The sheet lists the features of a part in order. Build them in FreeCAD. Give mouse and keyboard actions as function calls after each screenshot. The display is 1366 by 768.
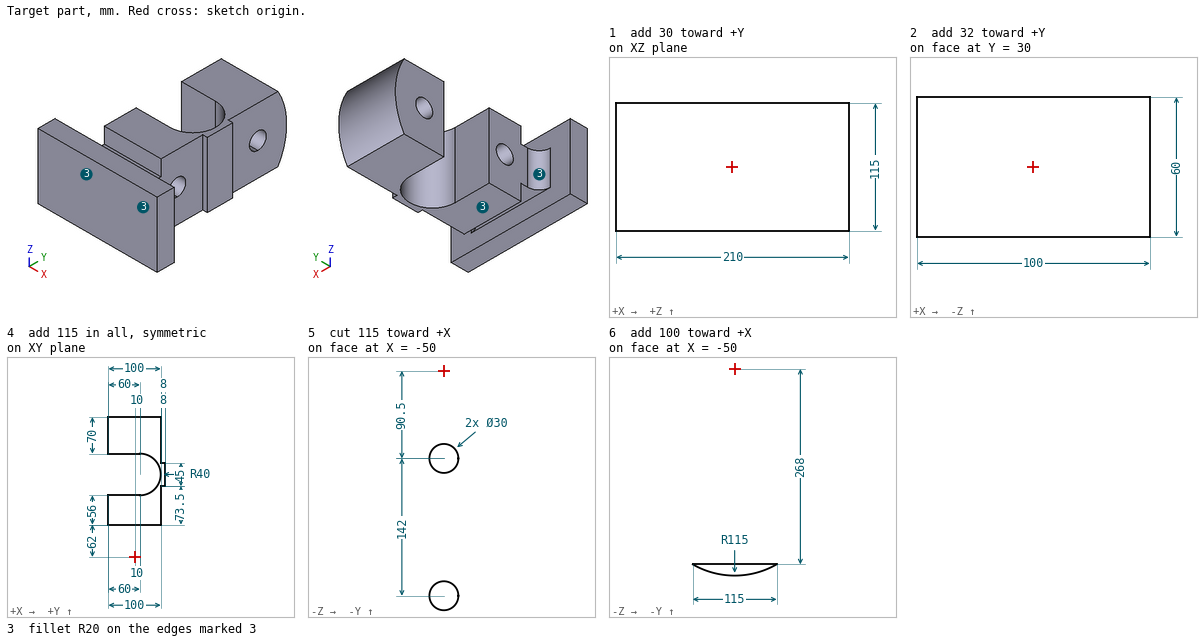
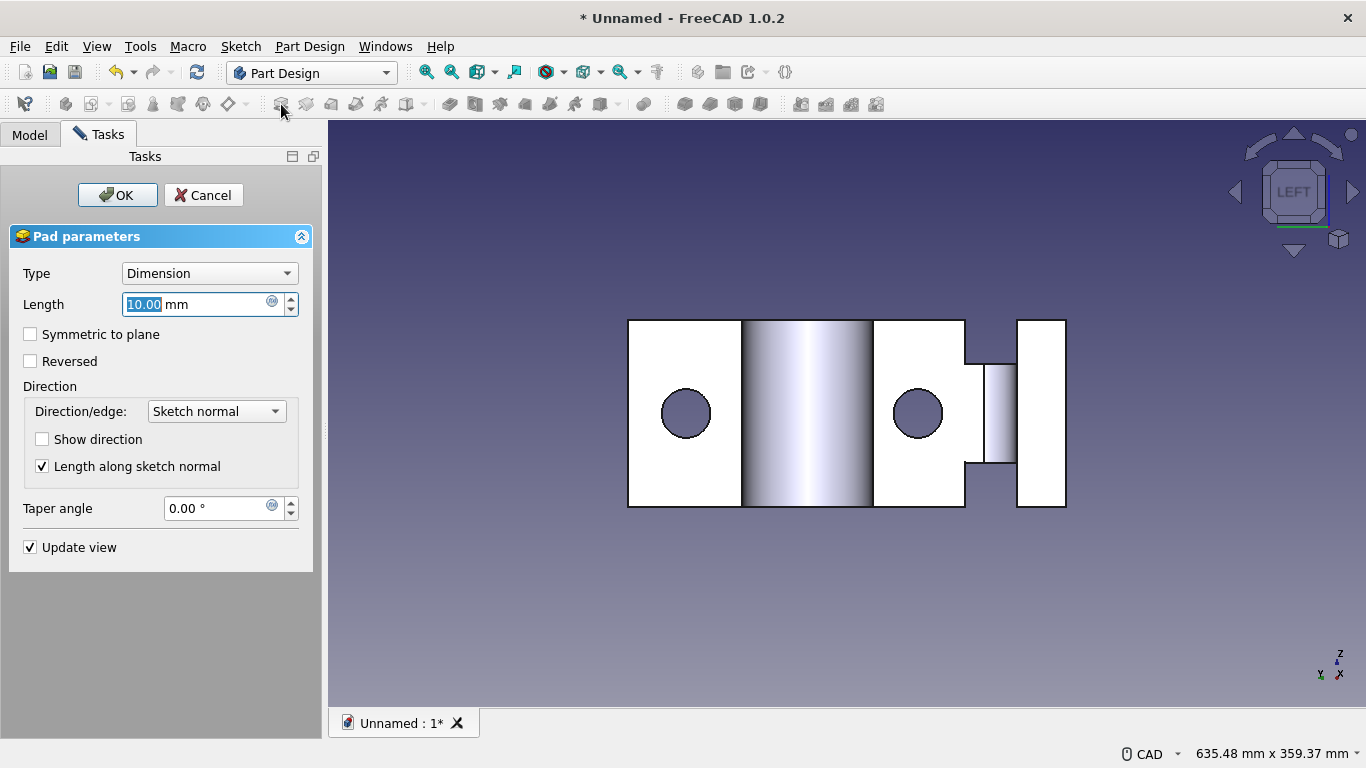
text(100)
key(Tab)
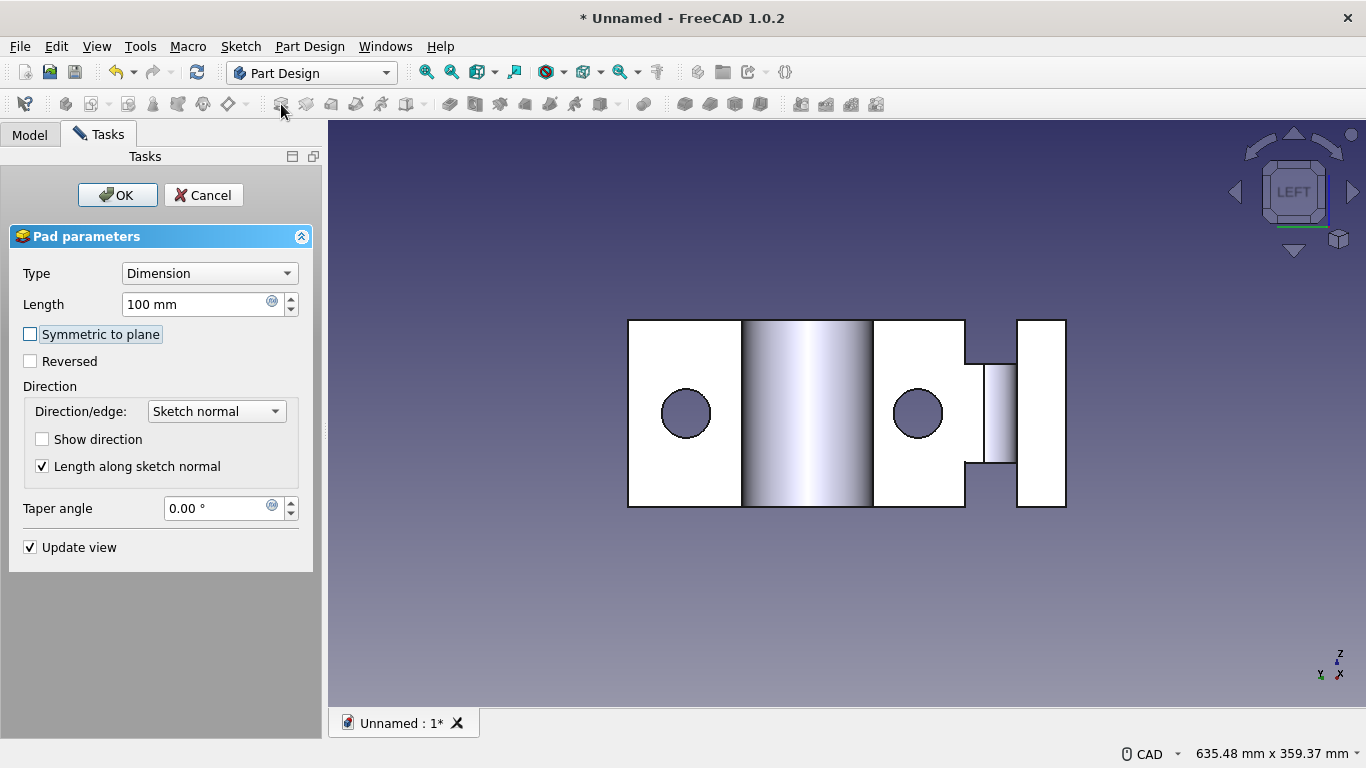
click(31, 361)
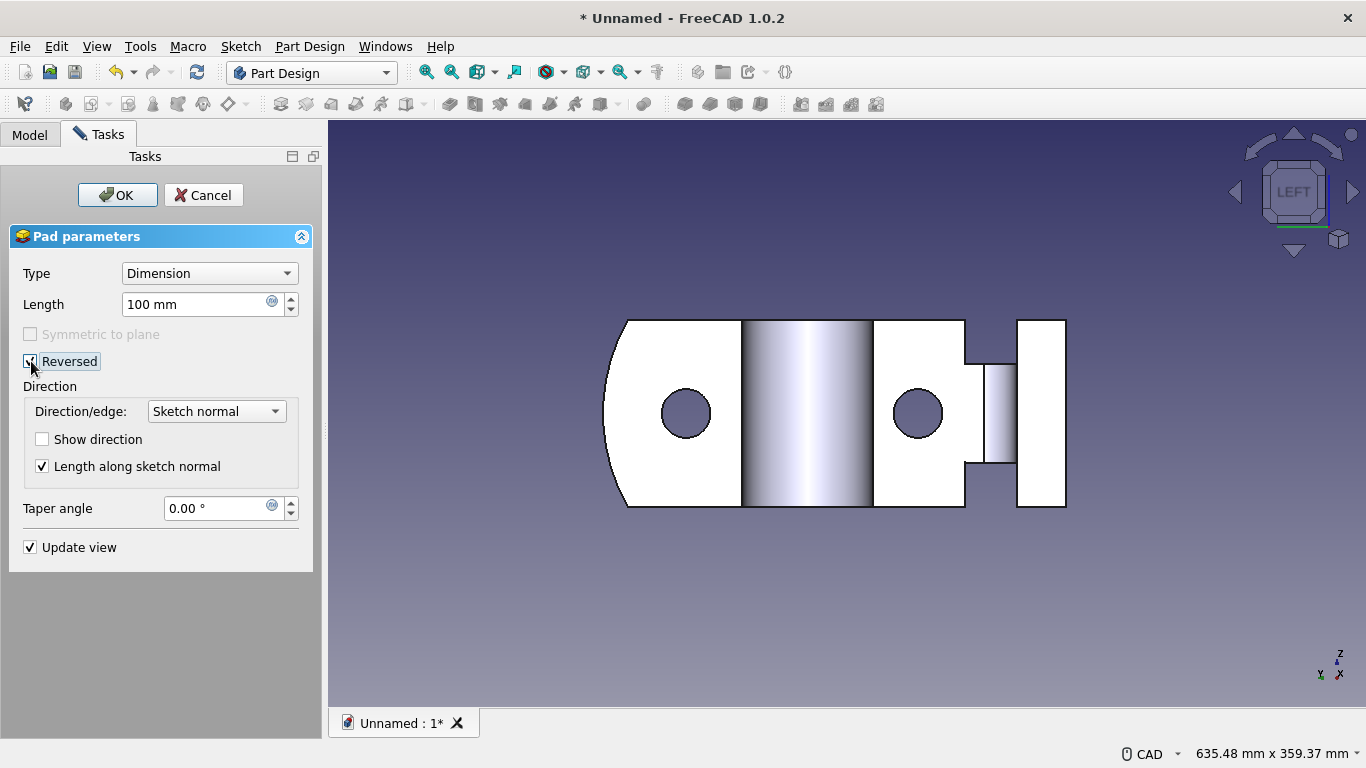
click(118, 195)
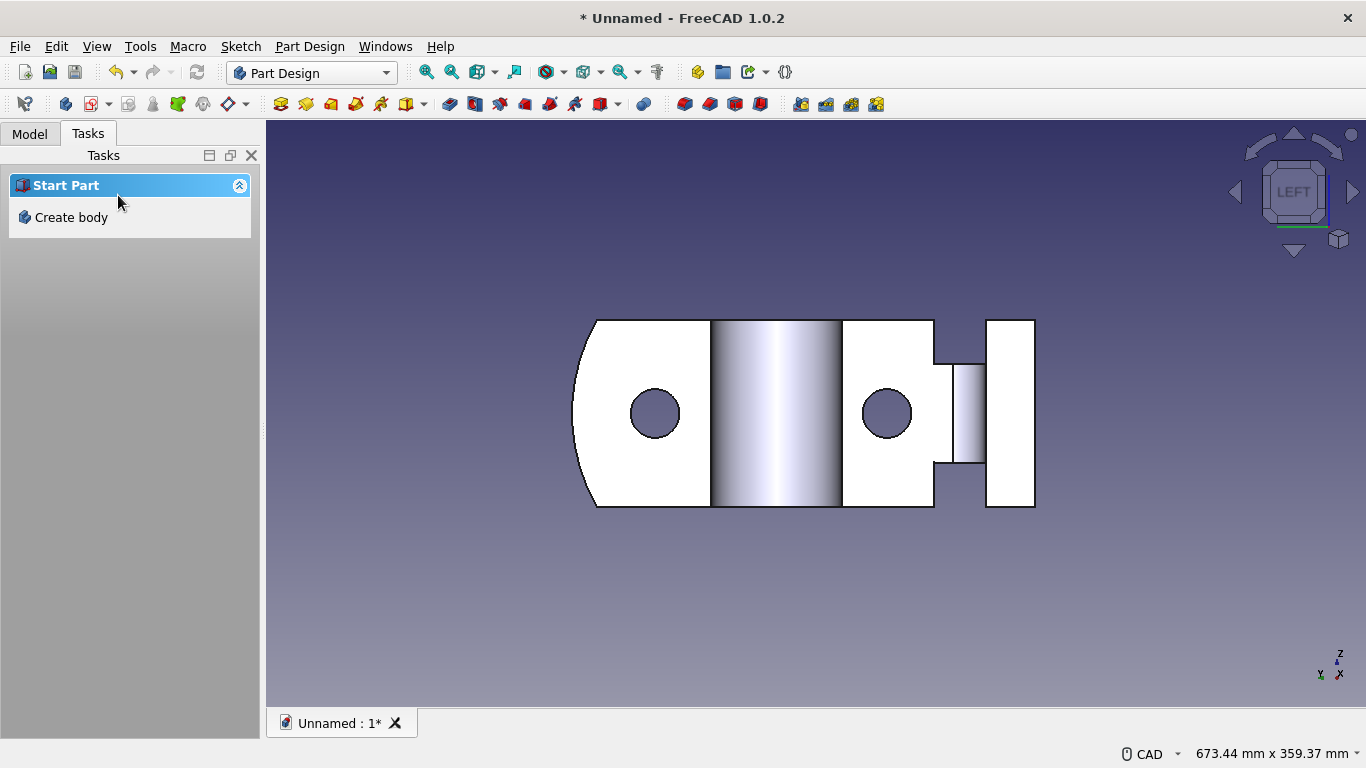
key(0)